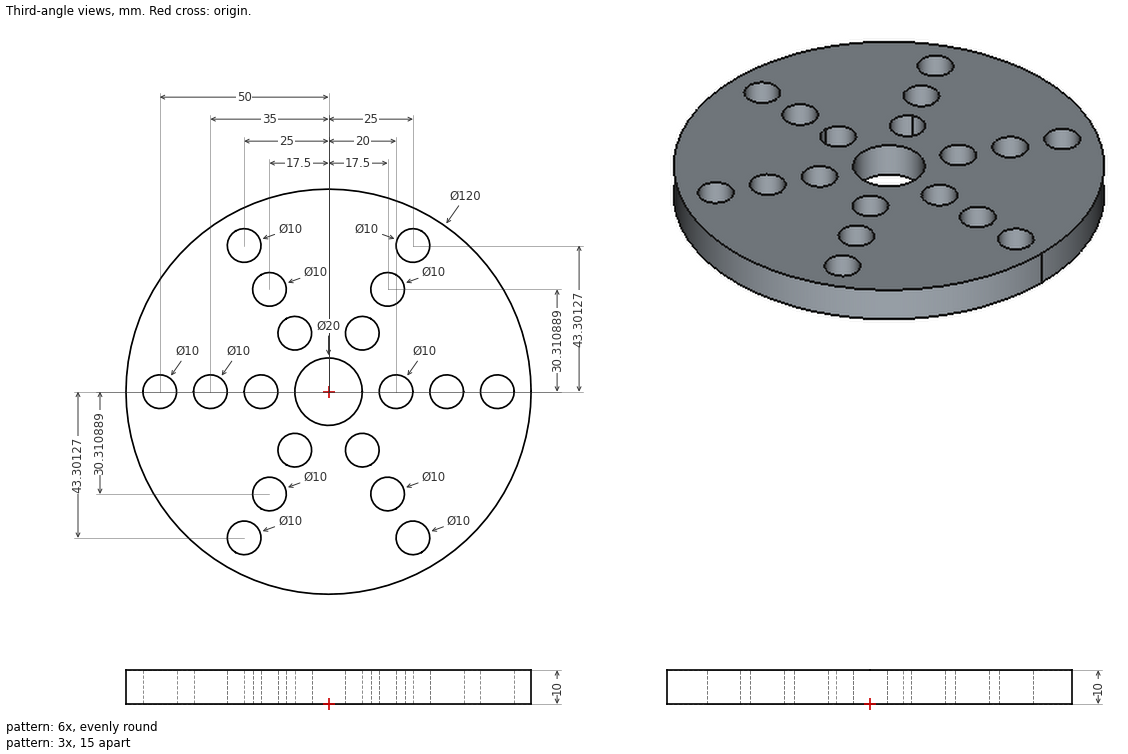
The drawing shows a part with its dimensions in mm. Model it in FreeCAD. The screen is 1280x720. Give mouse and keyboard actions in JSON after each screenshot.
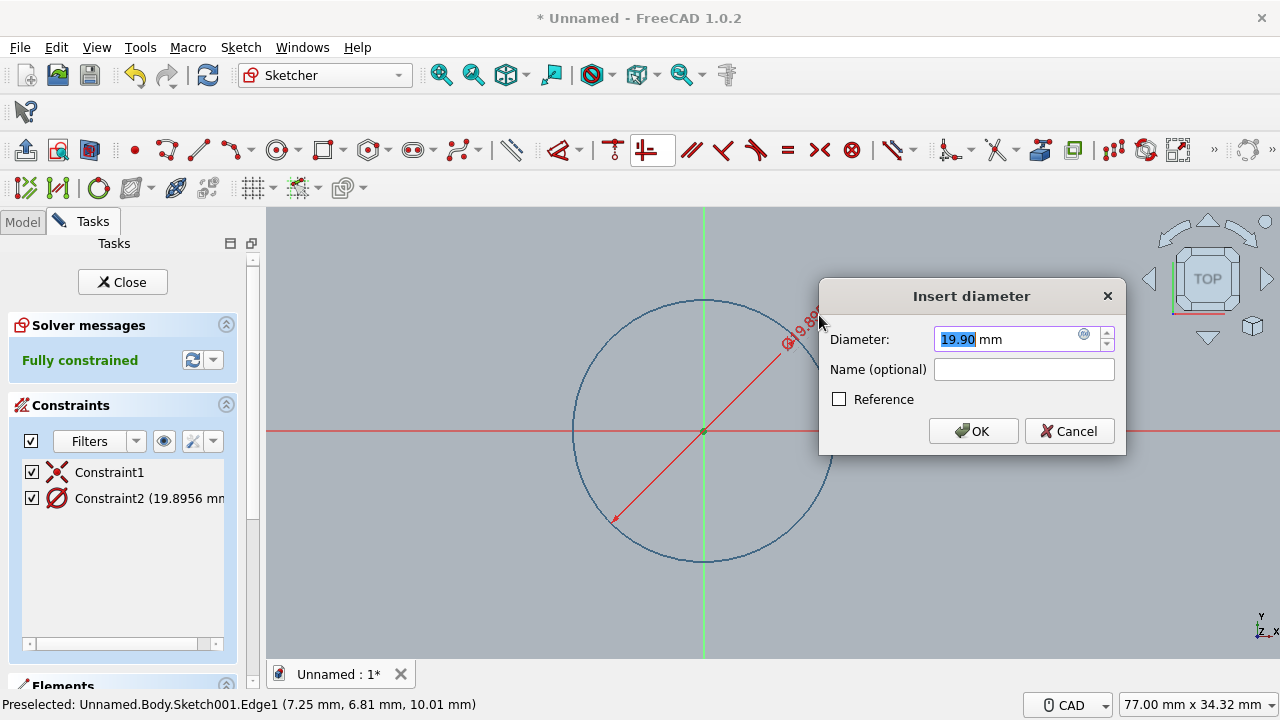
{"action": "type", "text": "20"}
{"action": "key", "text": "Return"}
{"action": "key", "text": "Escape"}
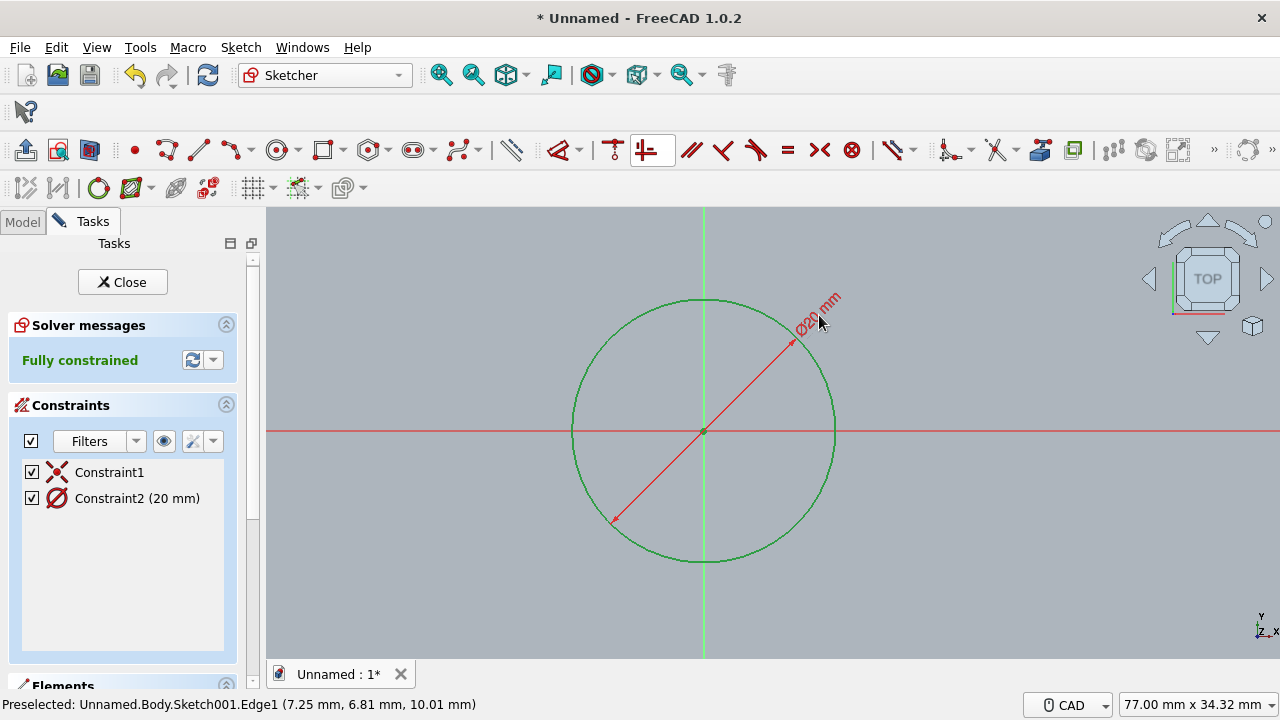
{"action": "left_click", "coordinate": [123, 282]}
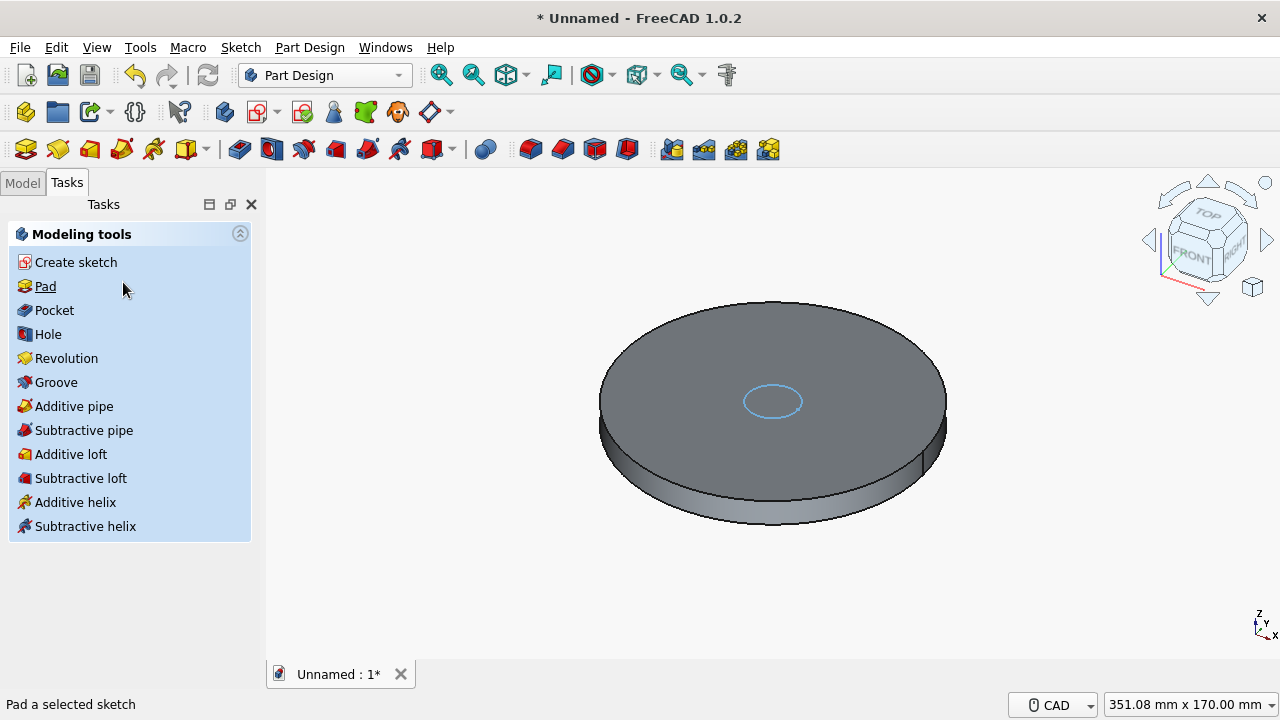
{"action": "left_click", "coordinate": [240, 150]}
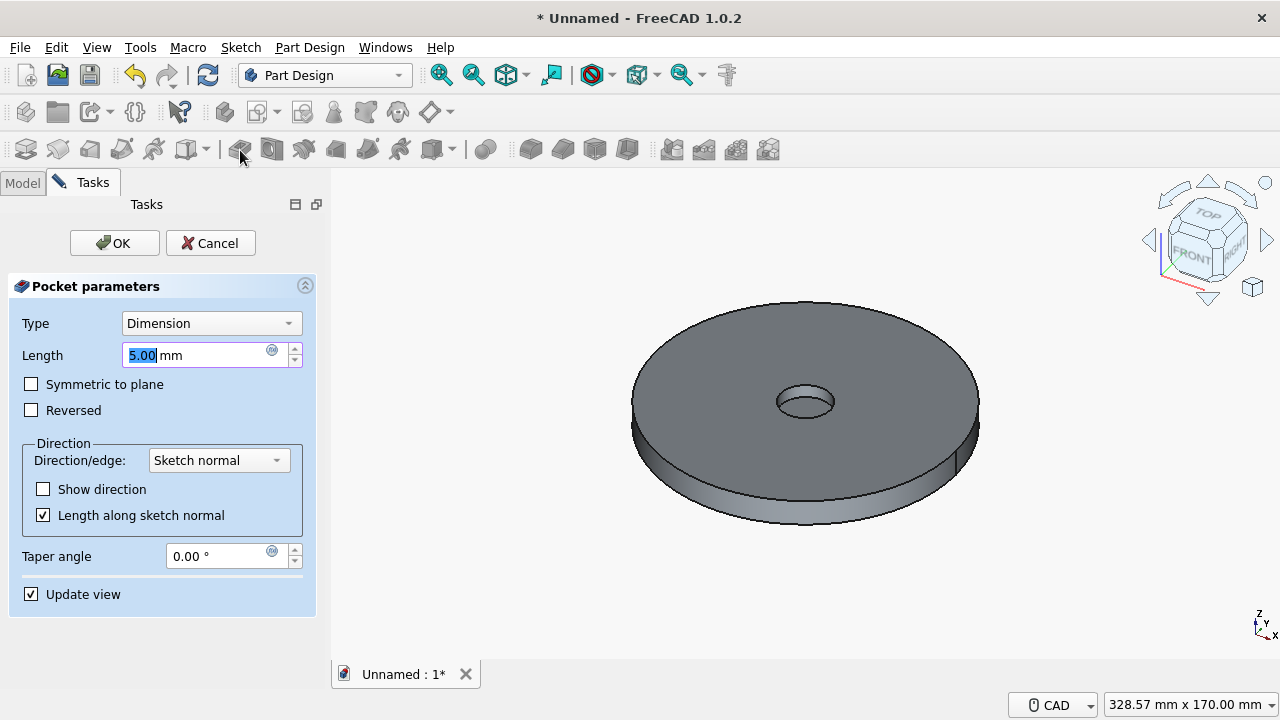
{"action": "type", "text": "10"}
{"action": "key", "text": "Tab"}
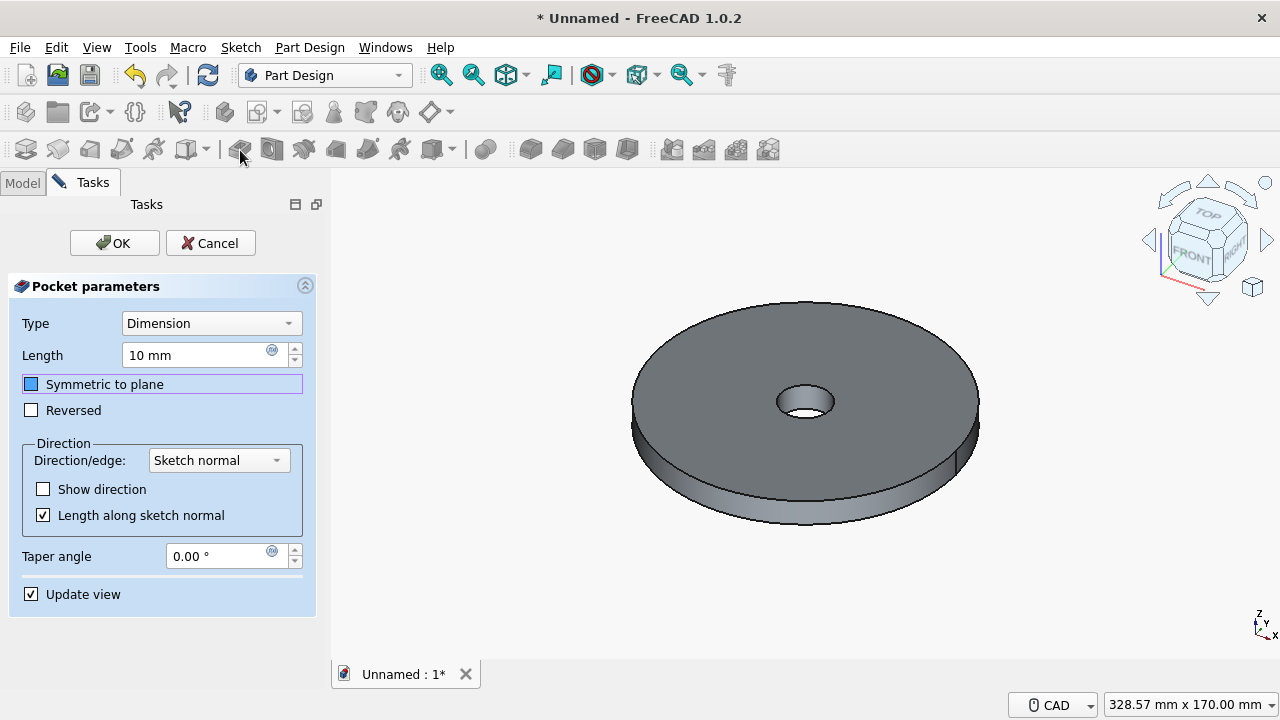
{"action": "left_click", "coordinate": [115, 243]}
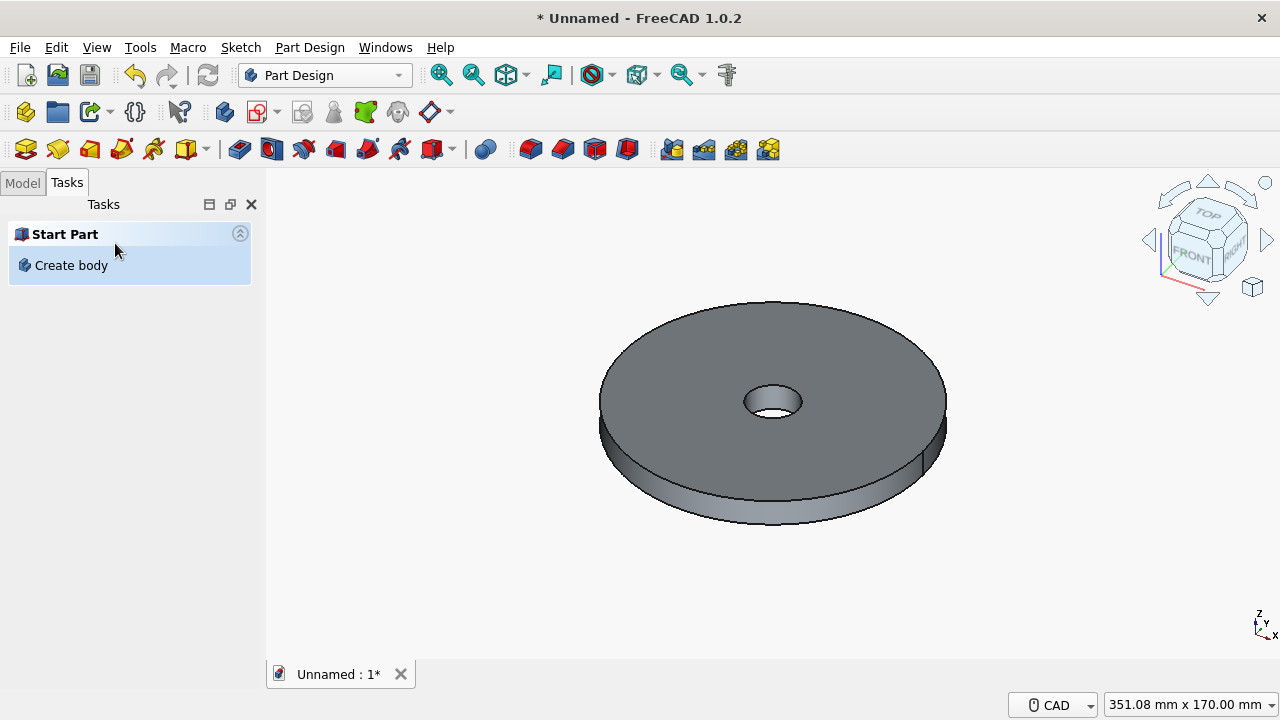
{"action": "left_click", "coordinate": [859, 429]}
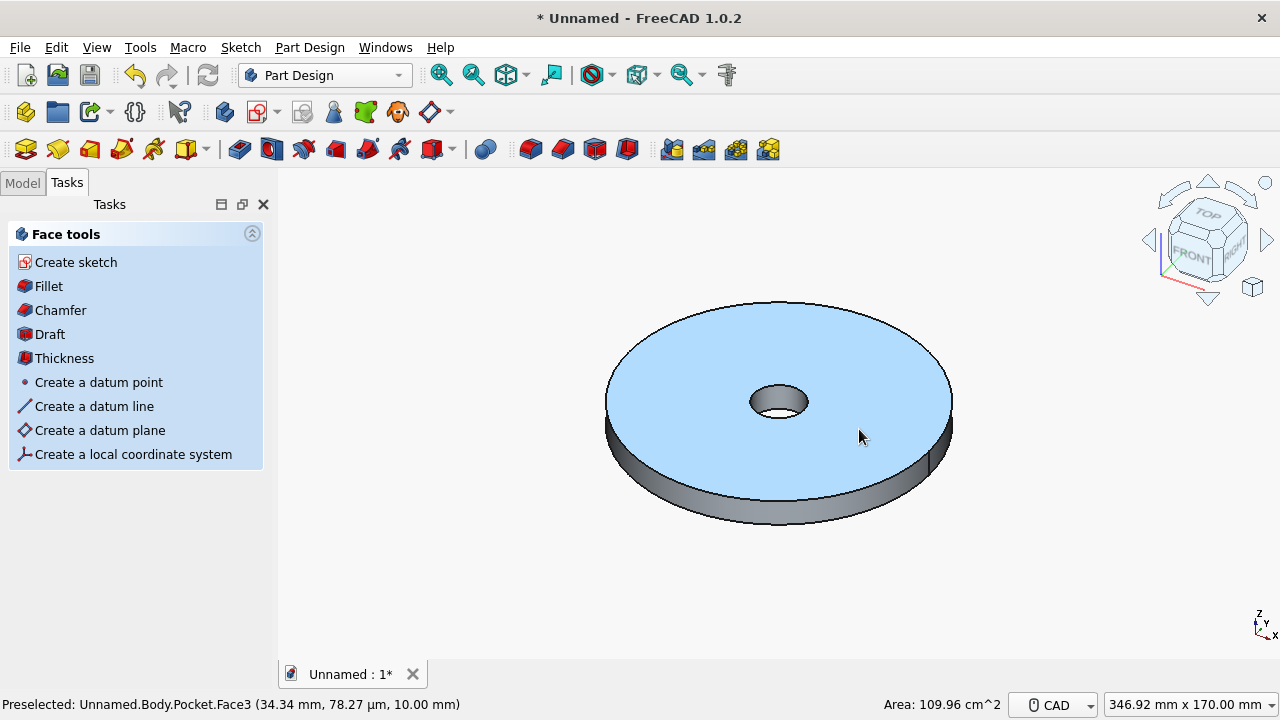
{"action": "left_click", "coordinate": [258, 112]}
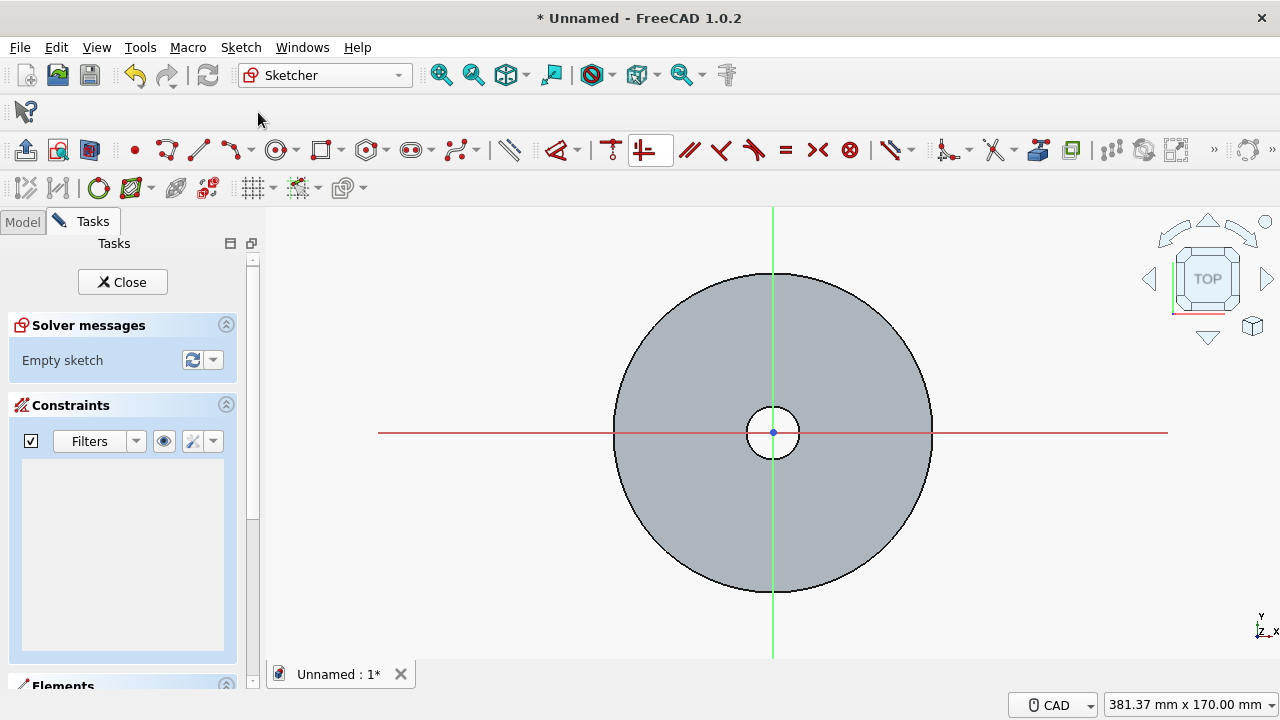
{"action": "scroll", "coordinate": [838, 433], "scroll_direction": "up", "scroll_amount": 12}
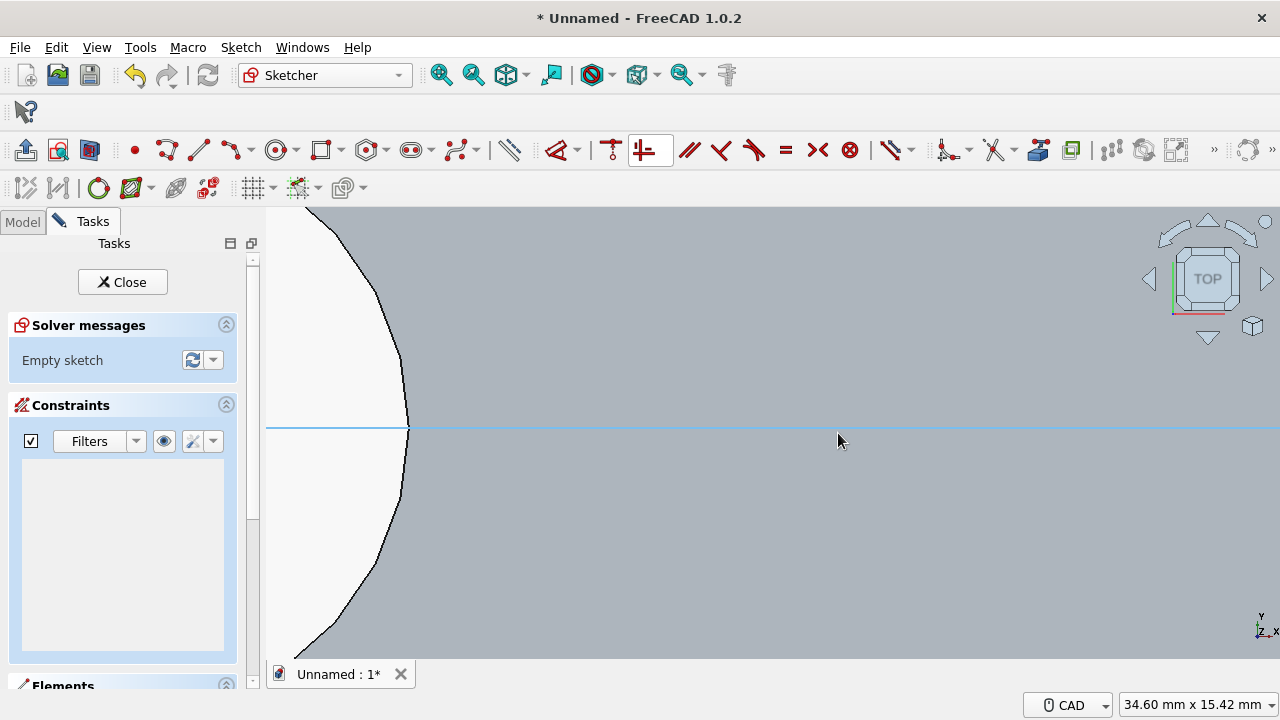
{"action": "left_click", "coordinate": [276, 150]}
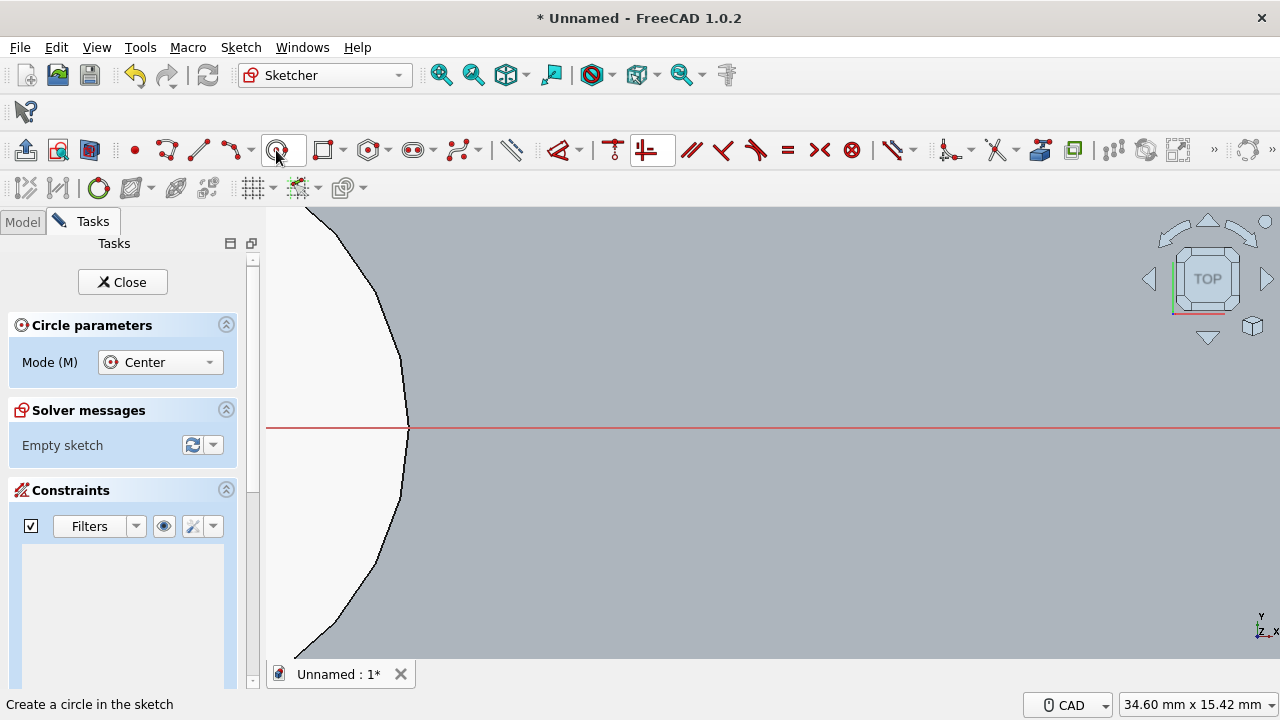
{"action": "left_click", "coordinate": [702, 428]}
{"action": "left_click", "coordinate": [806, 324]}
{"action": "key", "text": "Escape"}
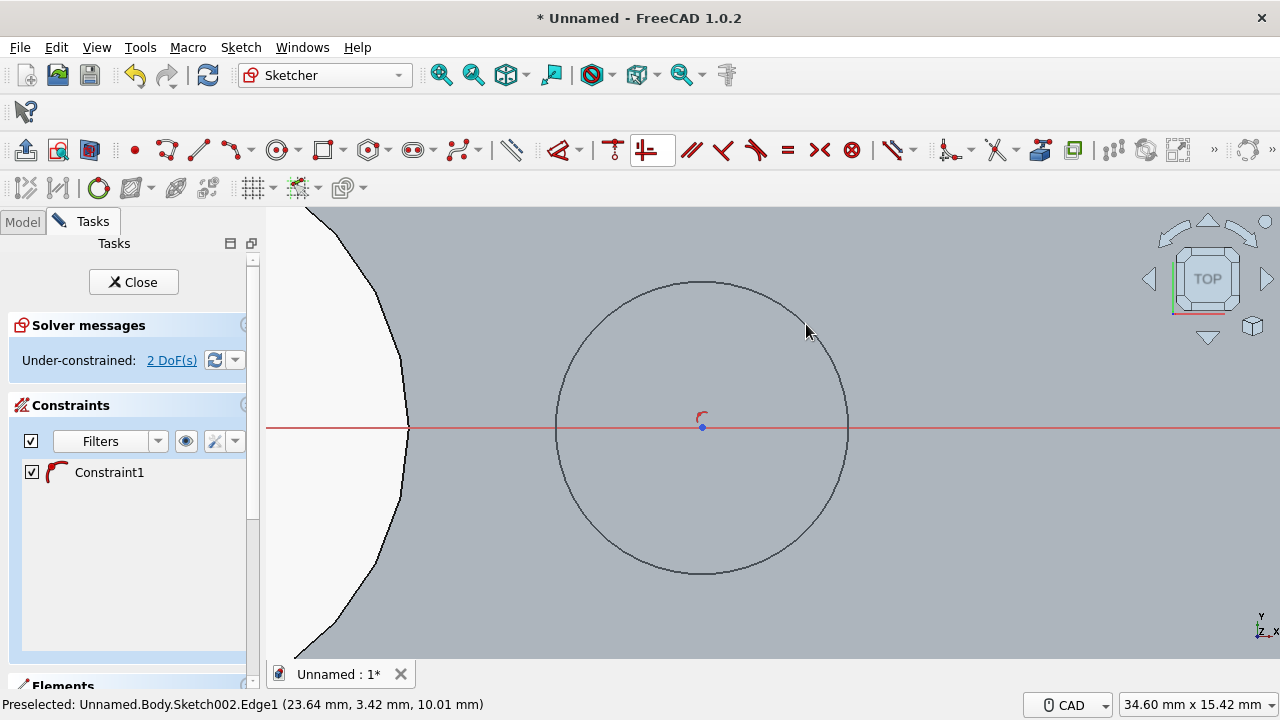
{"action": "left_click", "coordinate": [558, 150]}